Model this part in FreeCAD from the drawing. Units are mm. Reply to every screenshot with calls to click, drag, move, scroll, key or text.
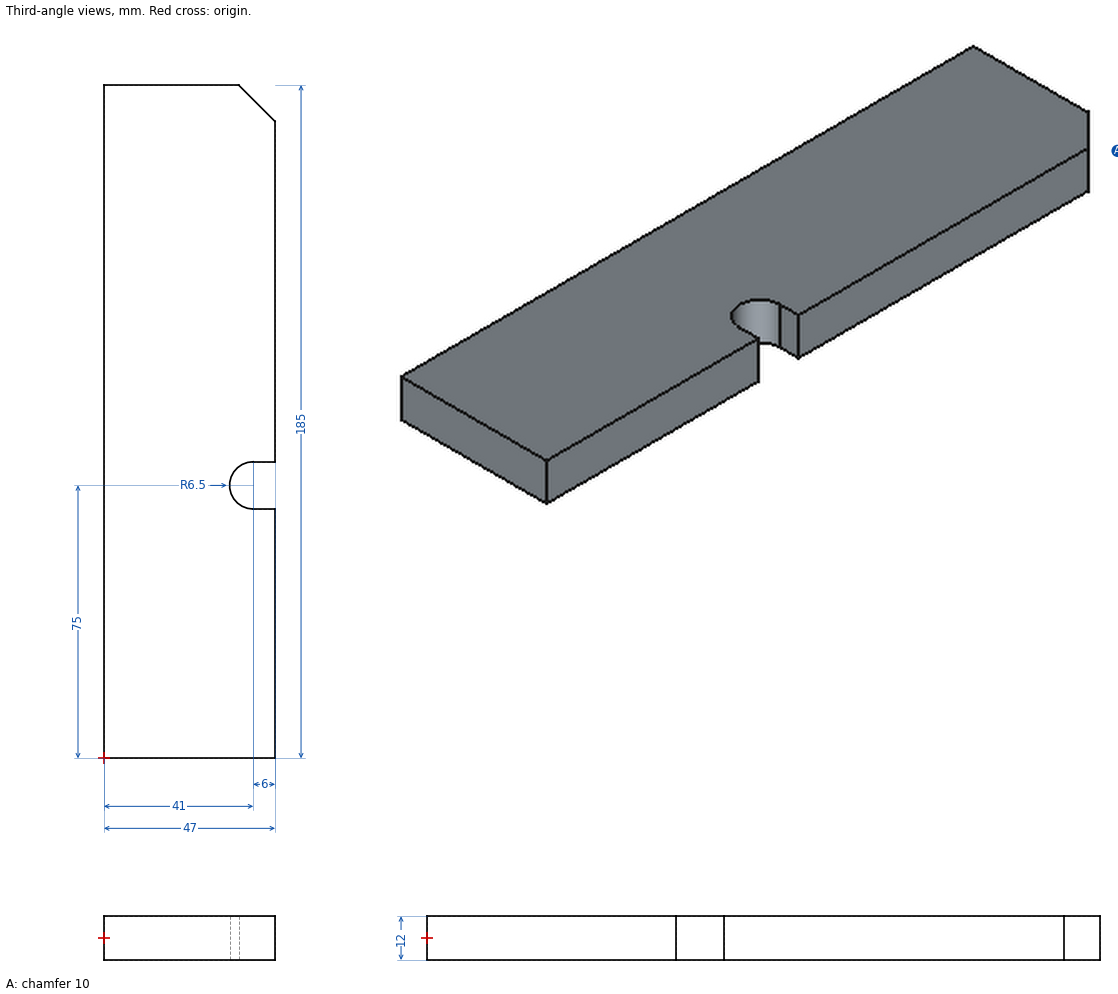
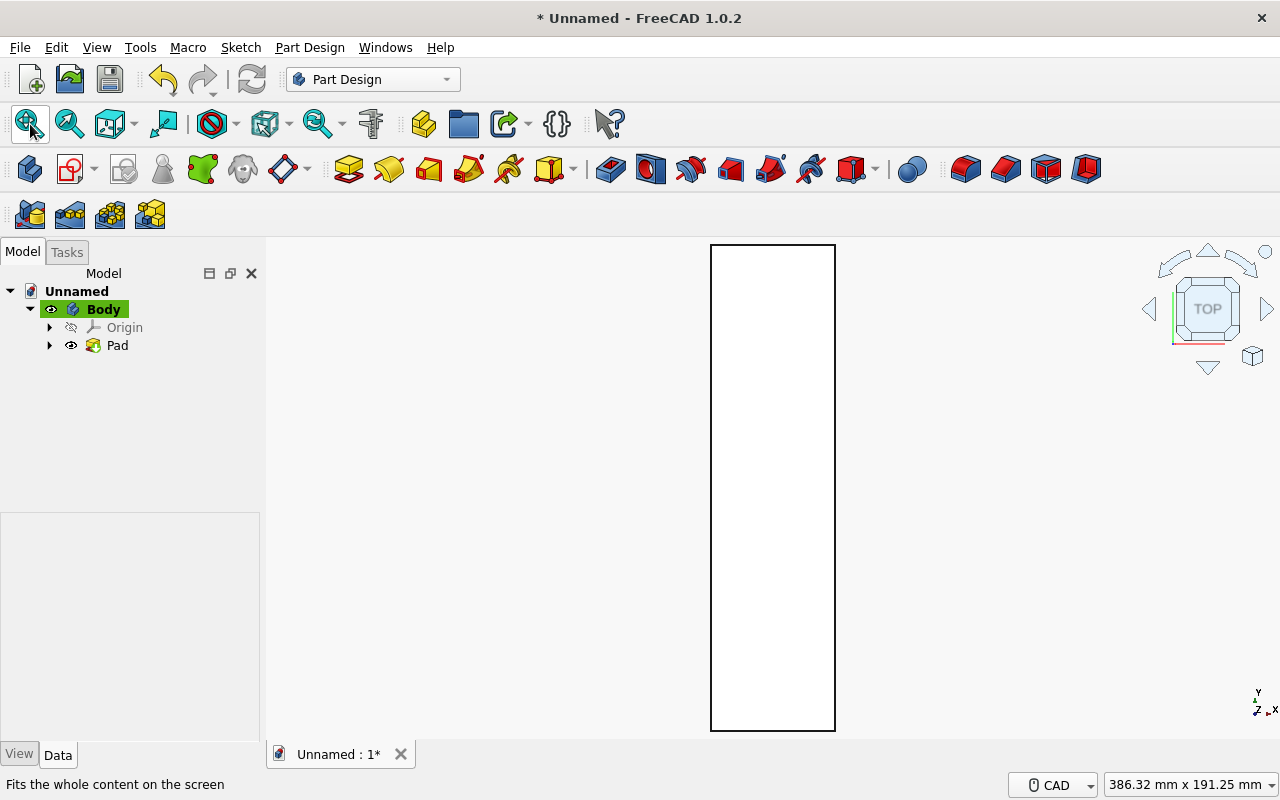
key(1)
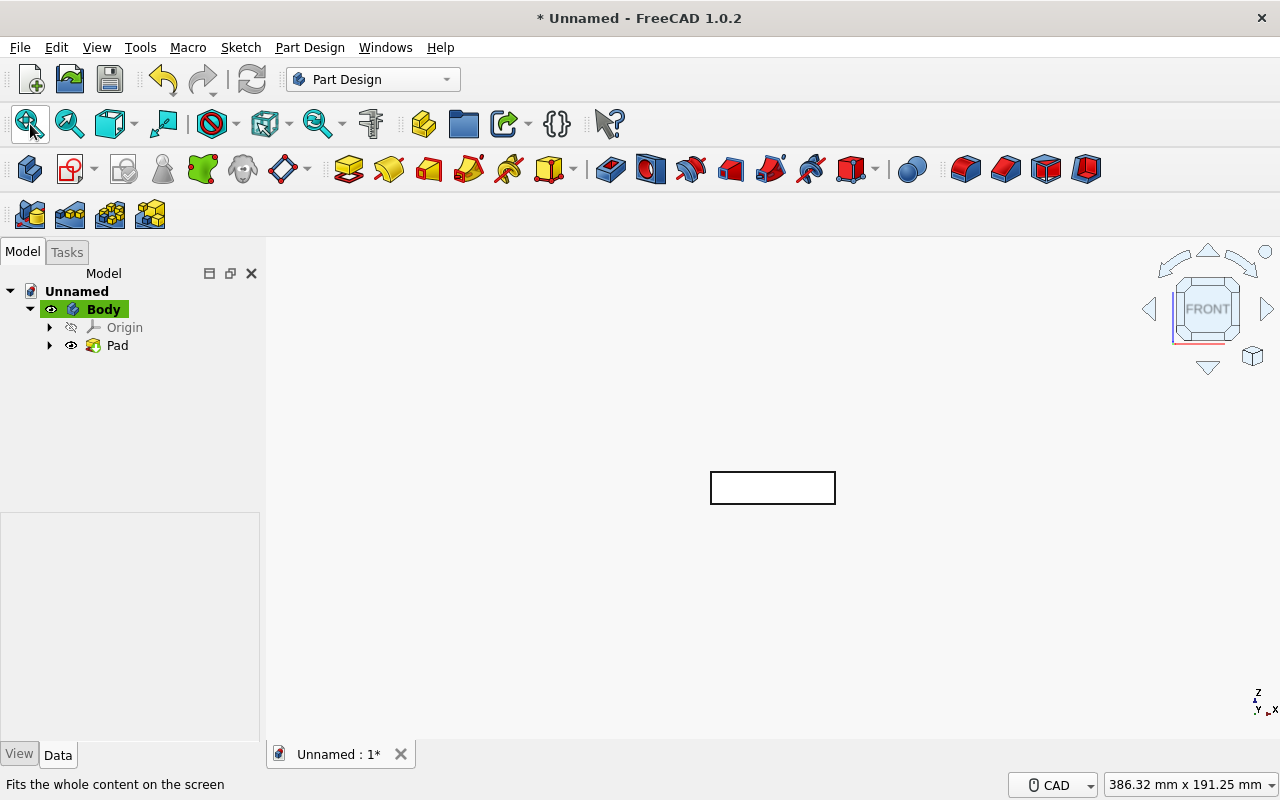
click(30, 124)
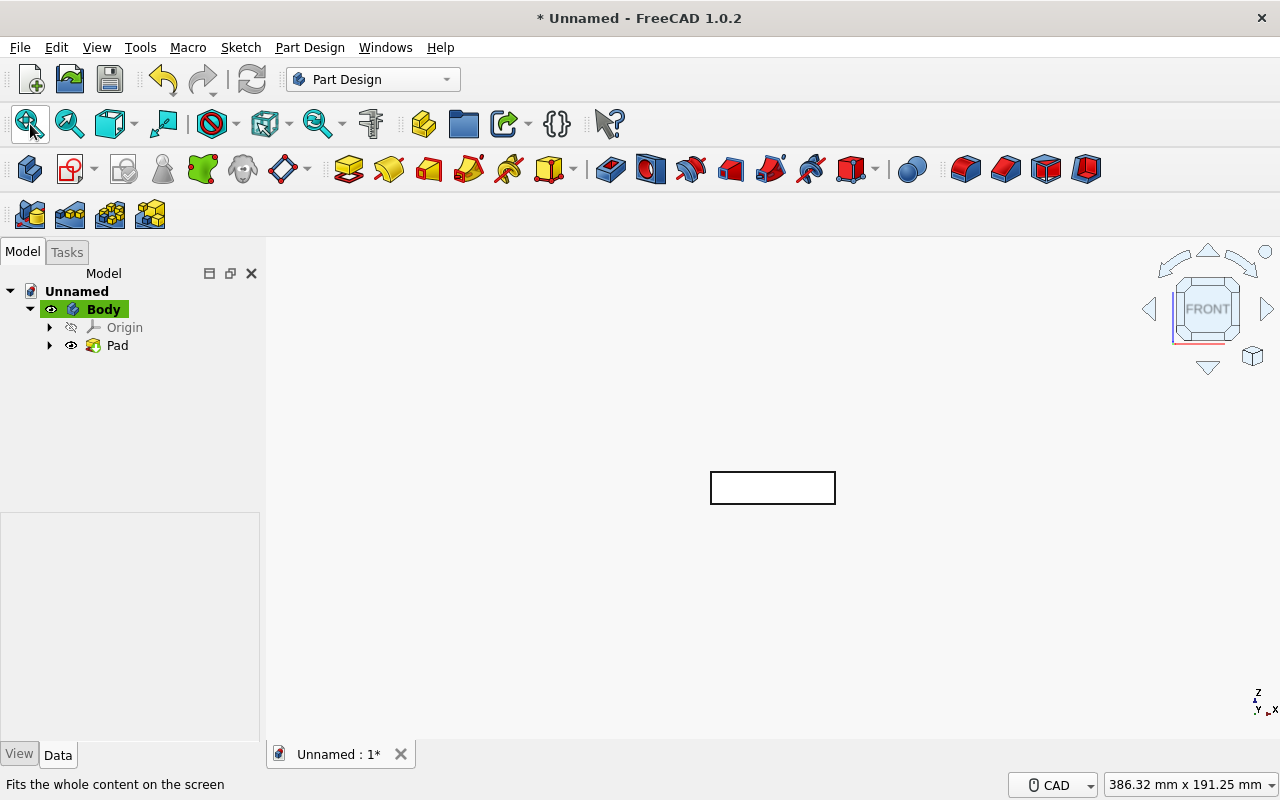
key(3)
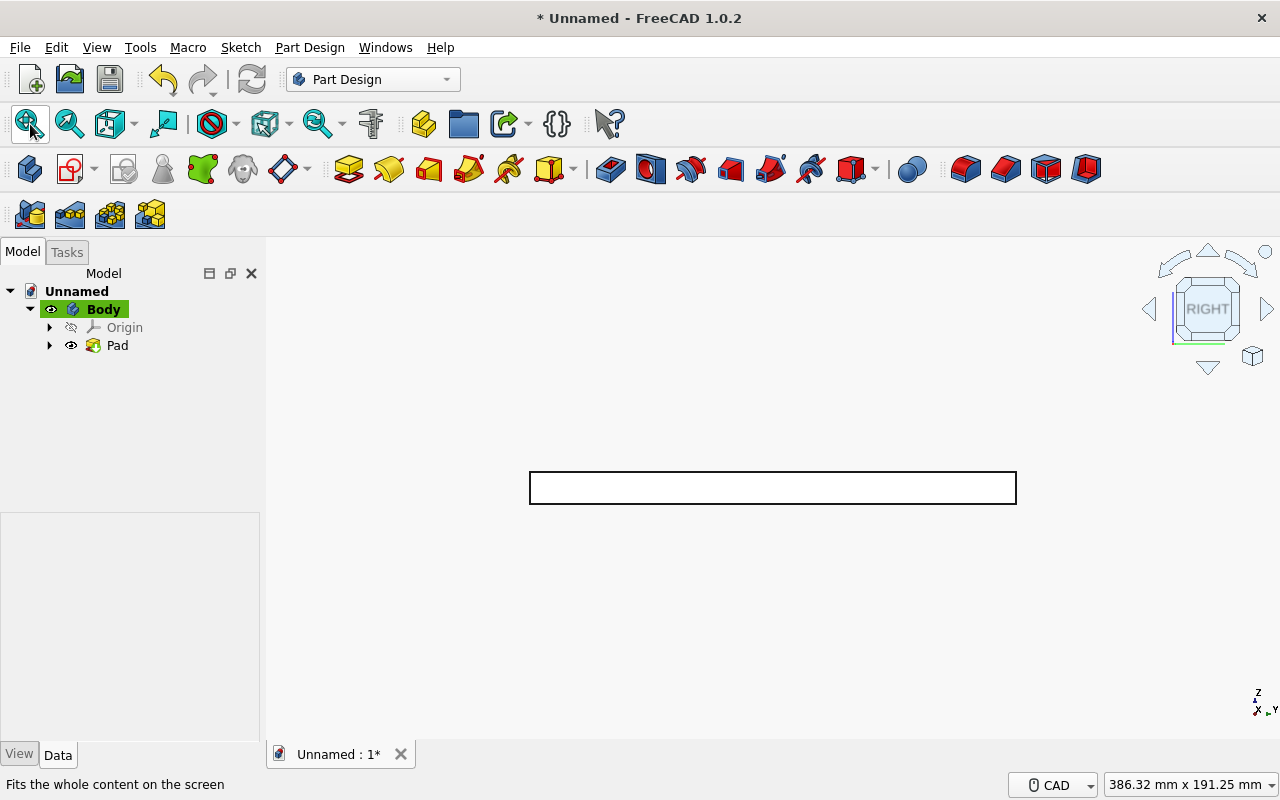
click(1016, 487)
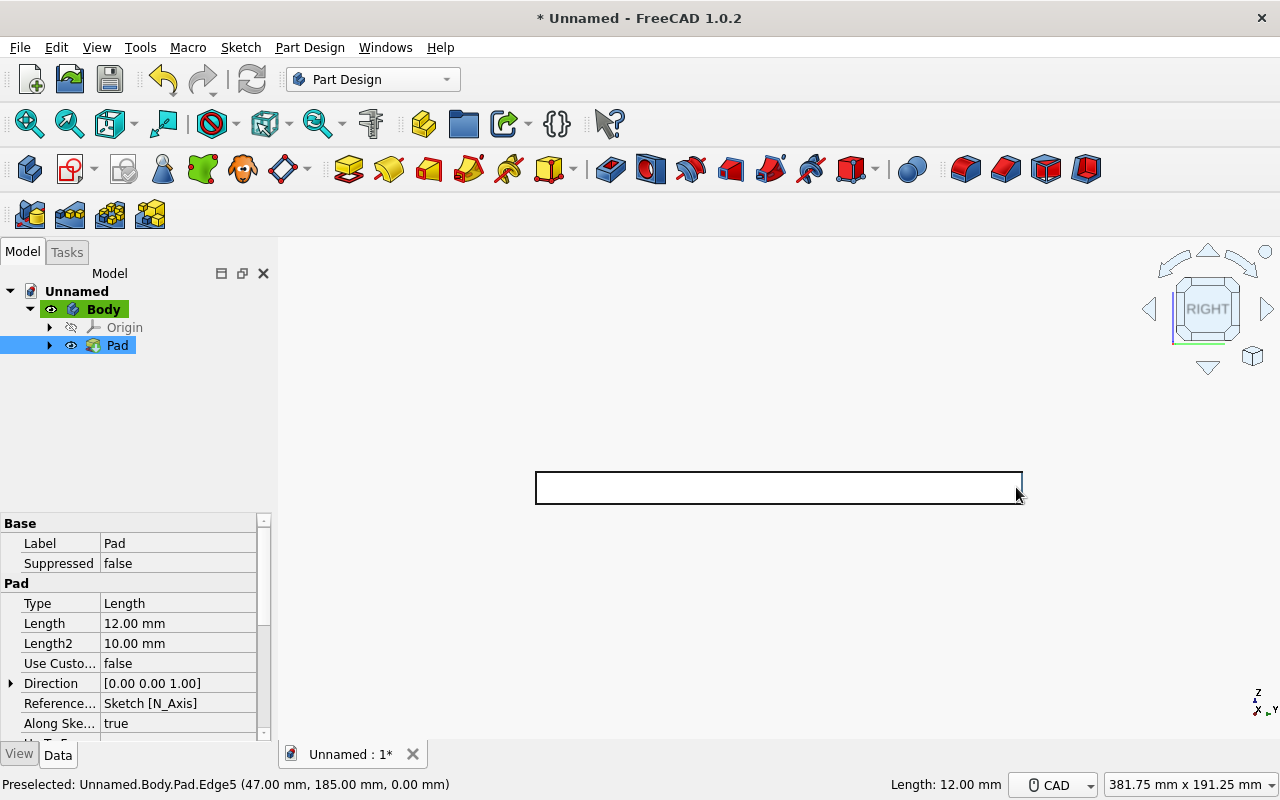
click(1006, 170)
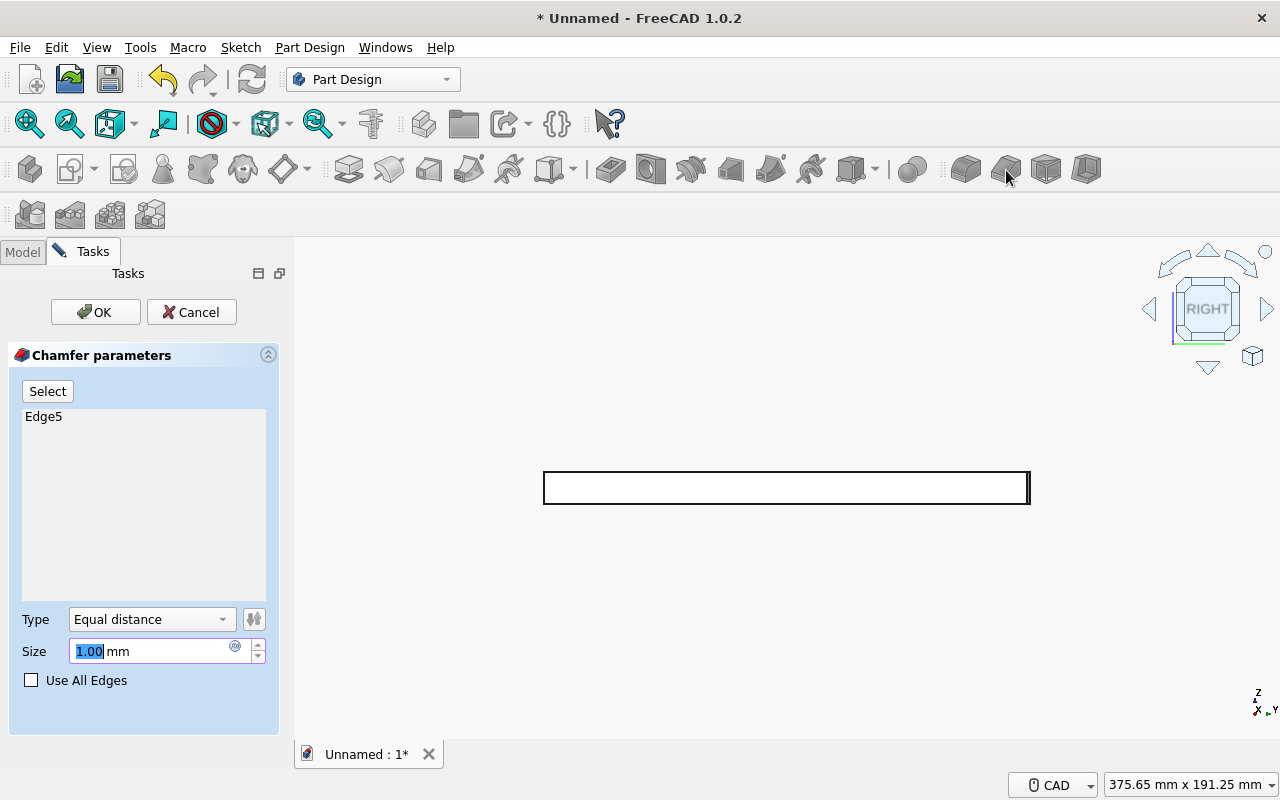
text(10)
key(Tab)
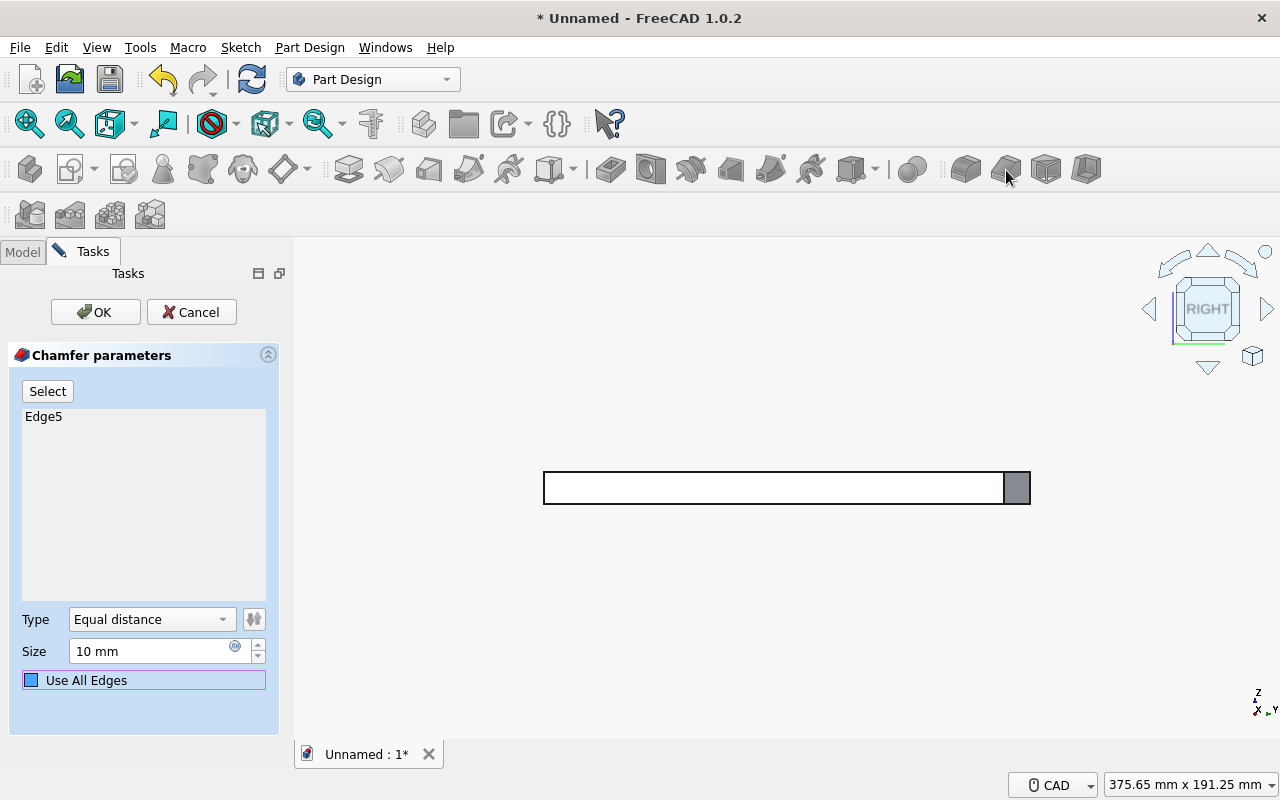
click(96, 312)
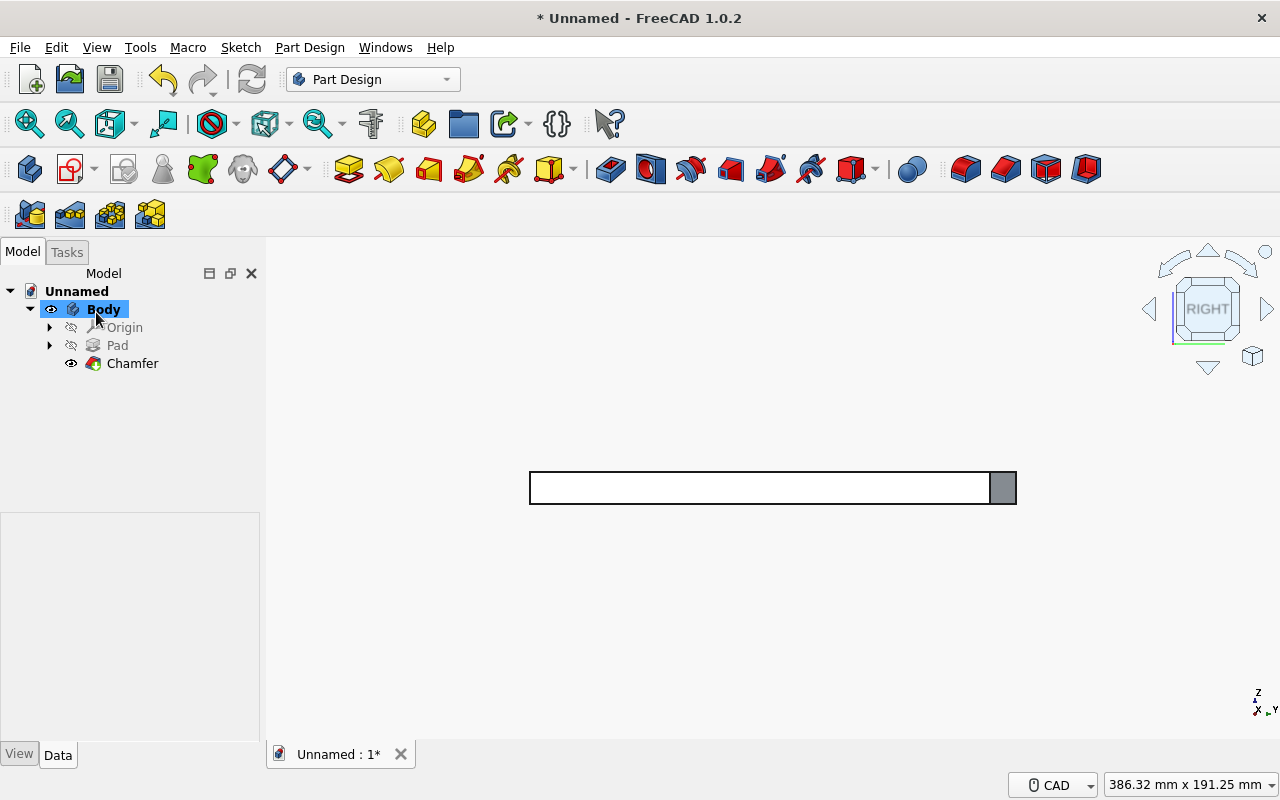
key(5)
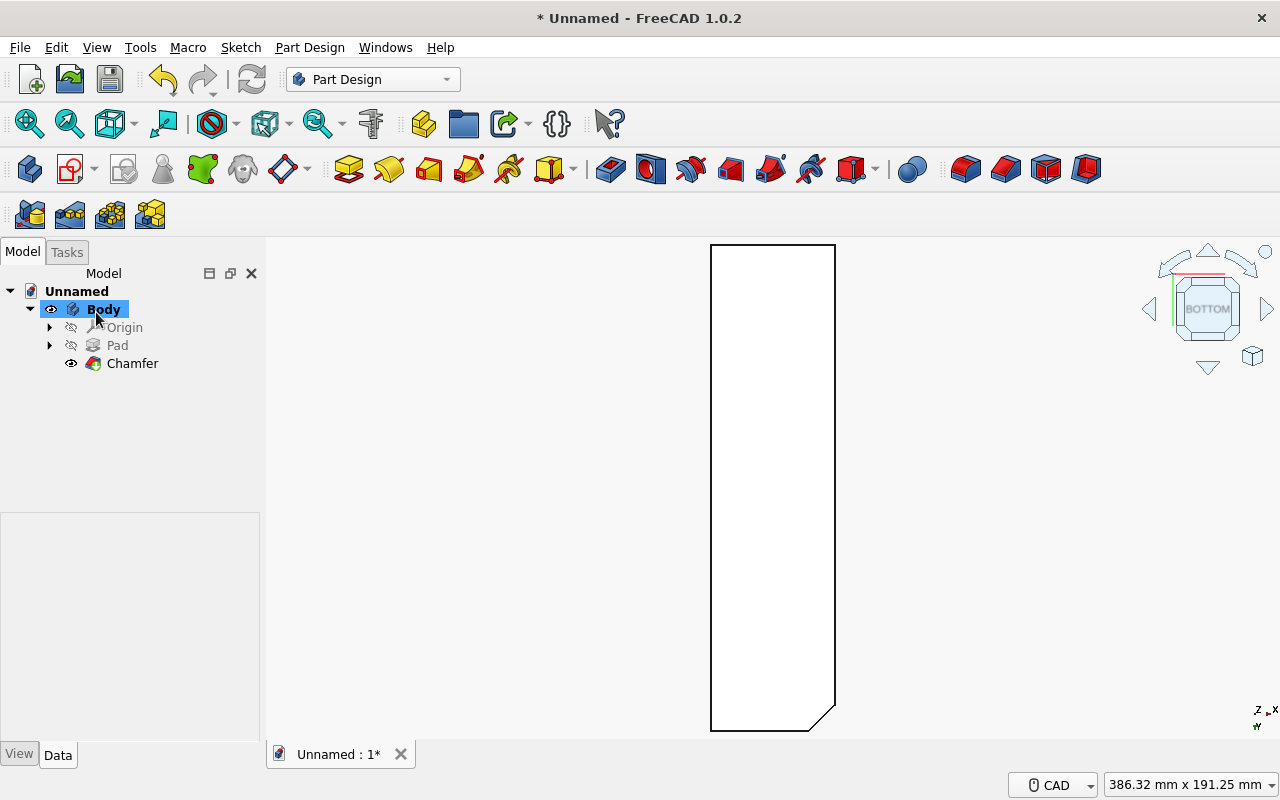
click(773, 626)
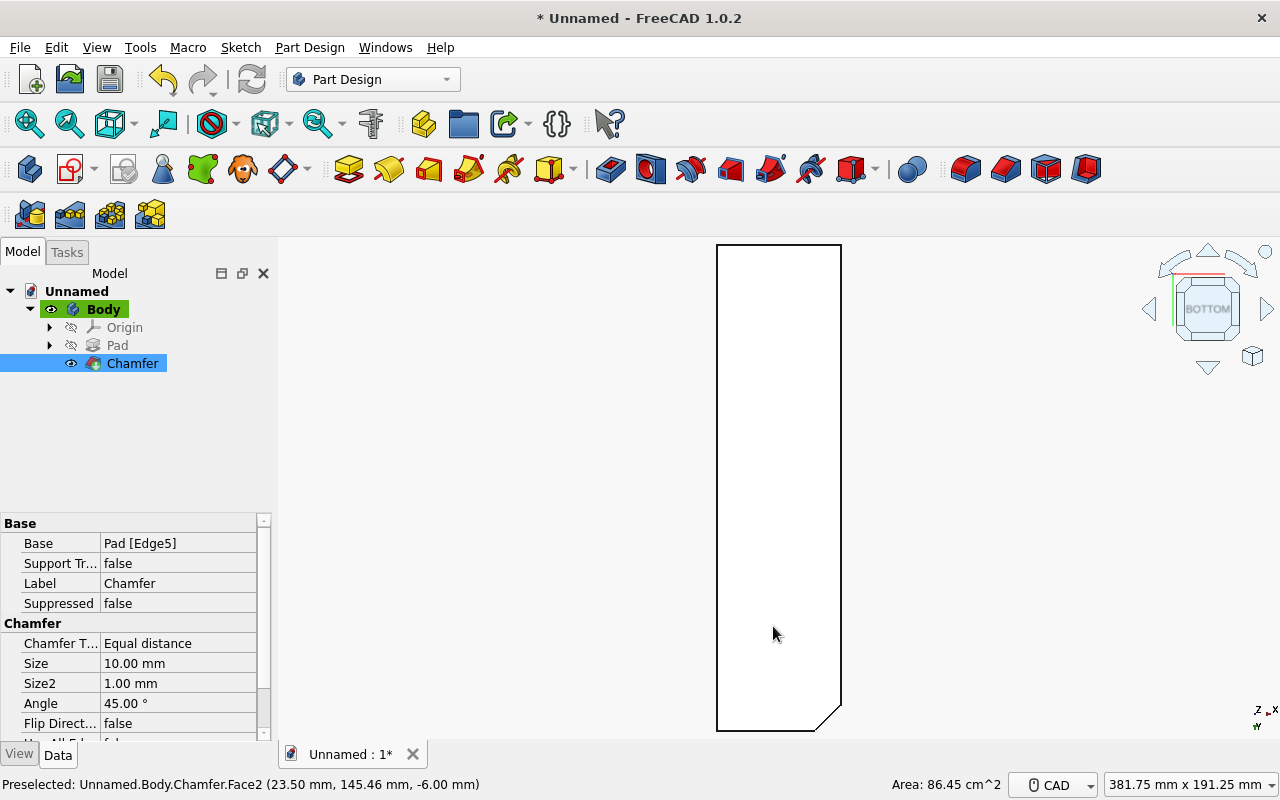
click(70, 170)